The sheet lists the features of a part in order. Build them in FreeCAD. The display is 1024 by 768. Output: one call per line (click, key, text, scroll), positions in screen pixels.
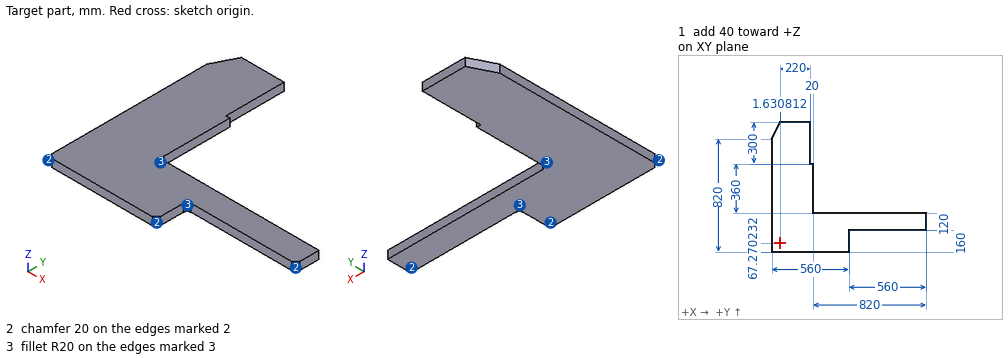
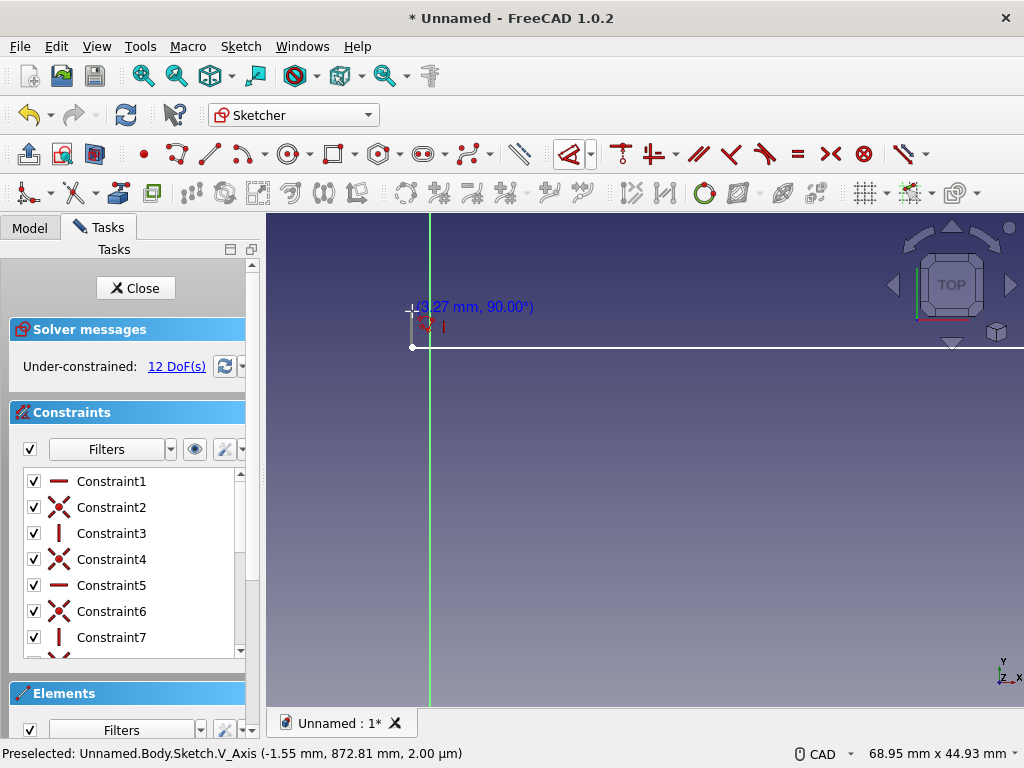
scroll(392, 287, down, 17)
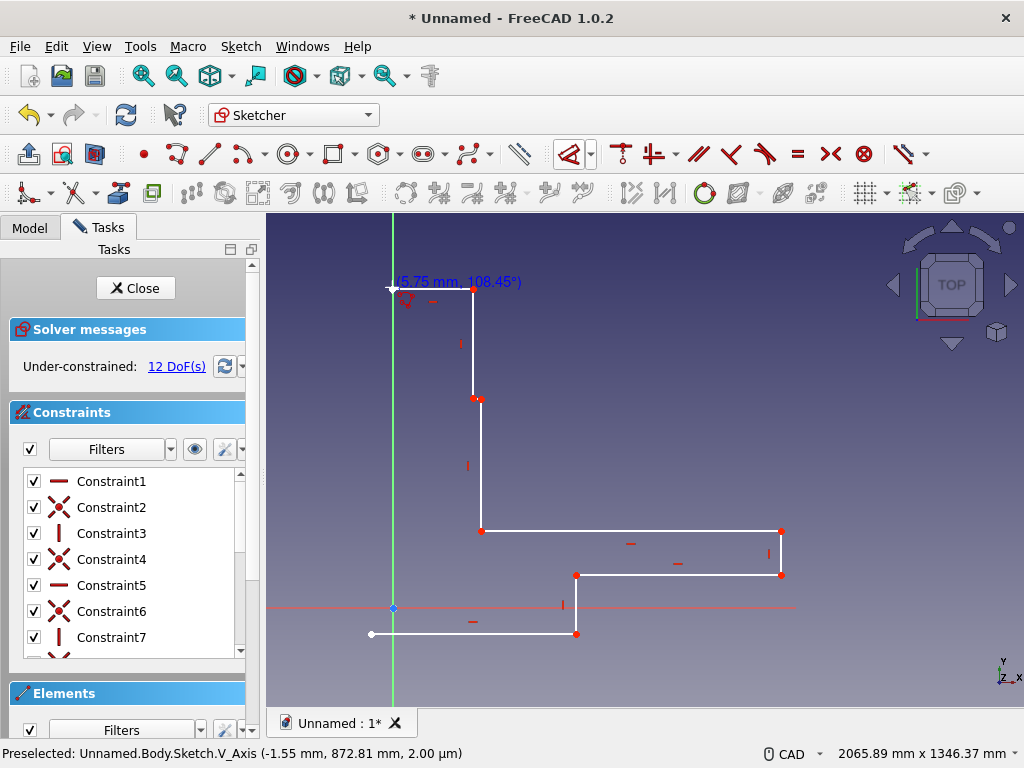
click(371, 332)
click(371, 634)
key(Escape)
key(Escape)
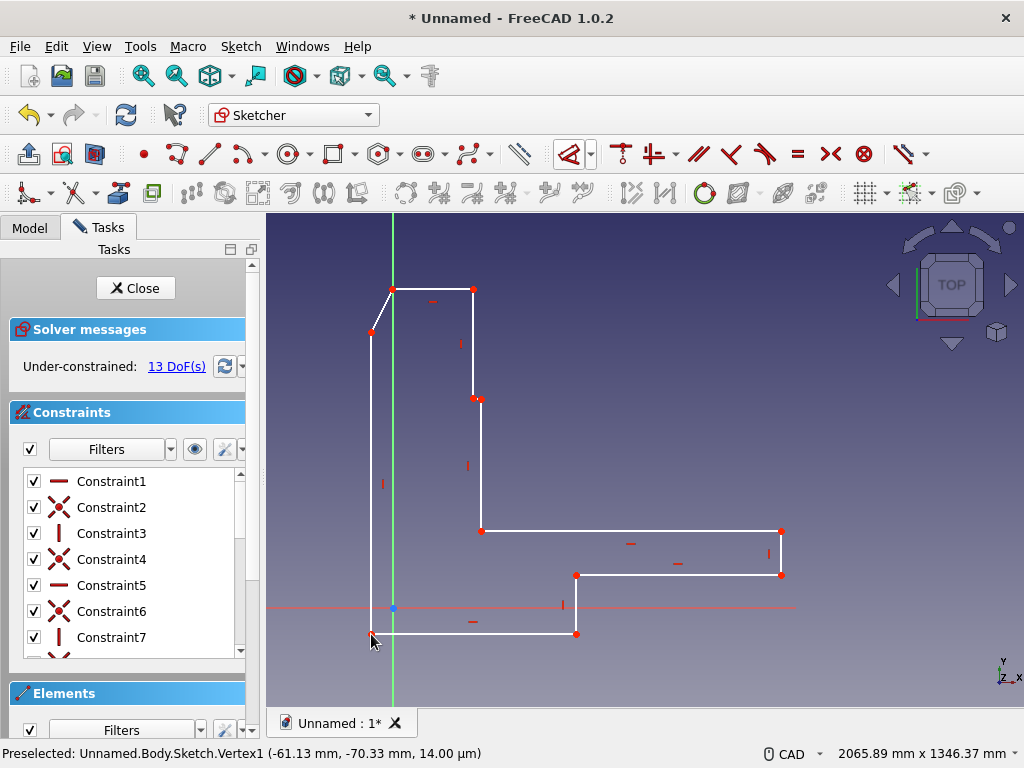
scroll(477, 399, up, 7)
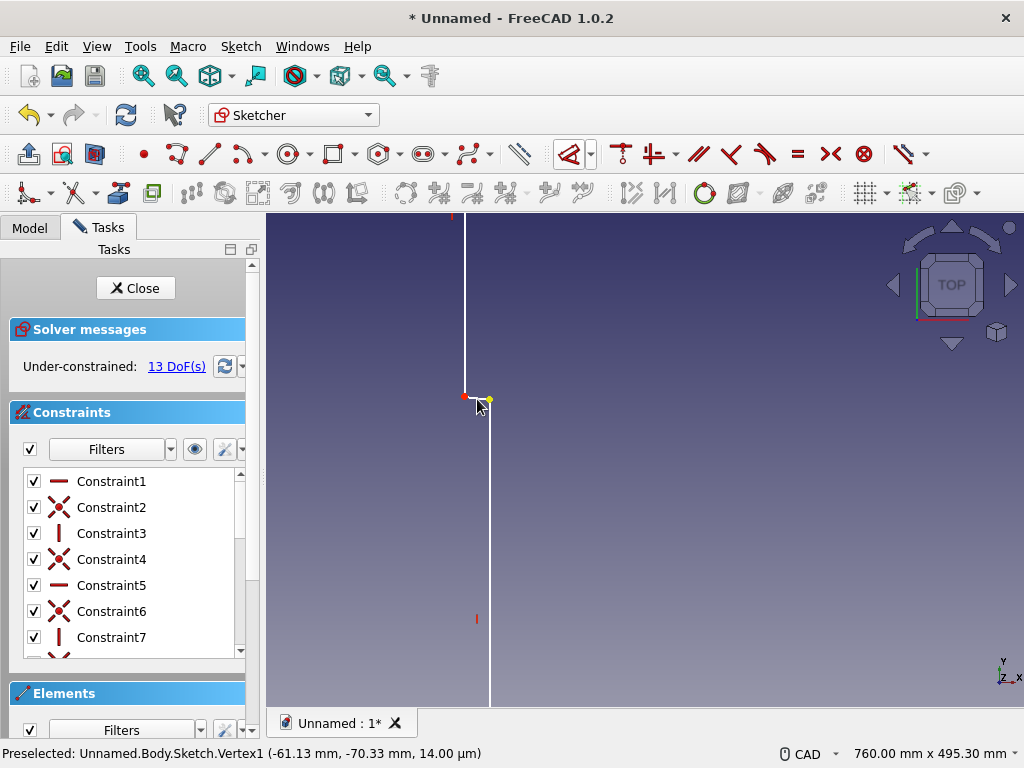
click(477, 398)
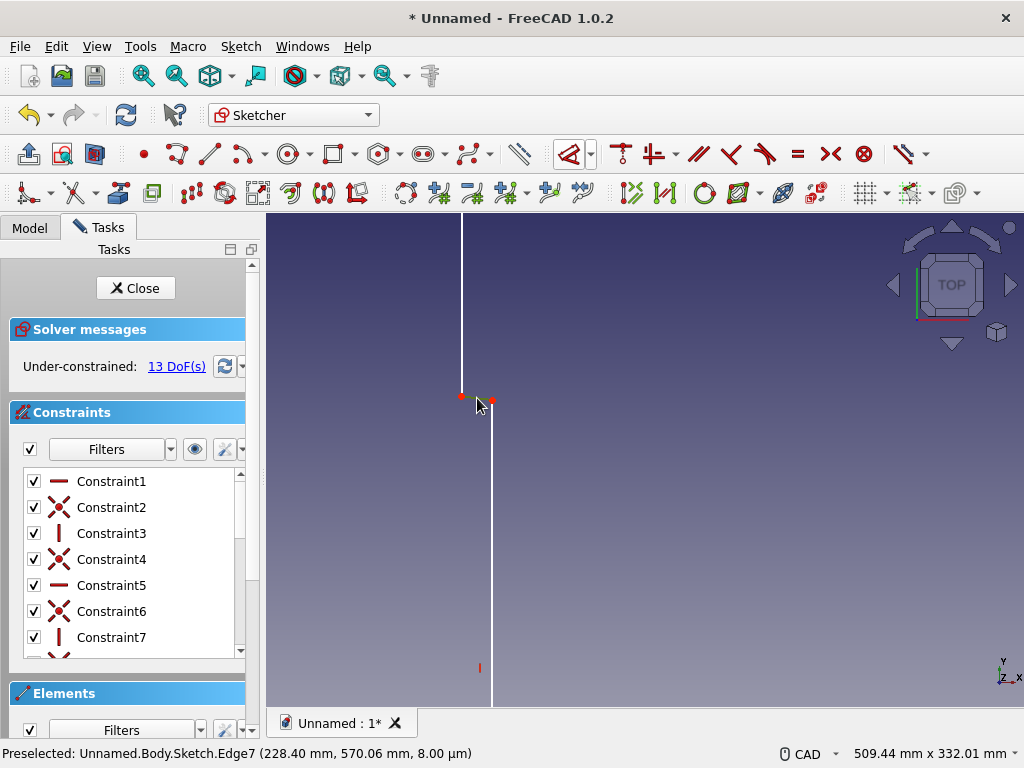
key(h)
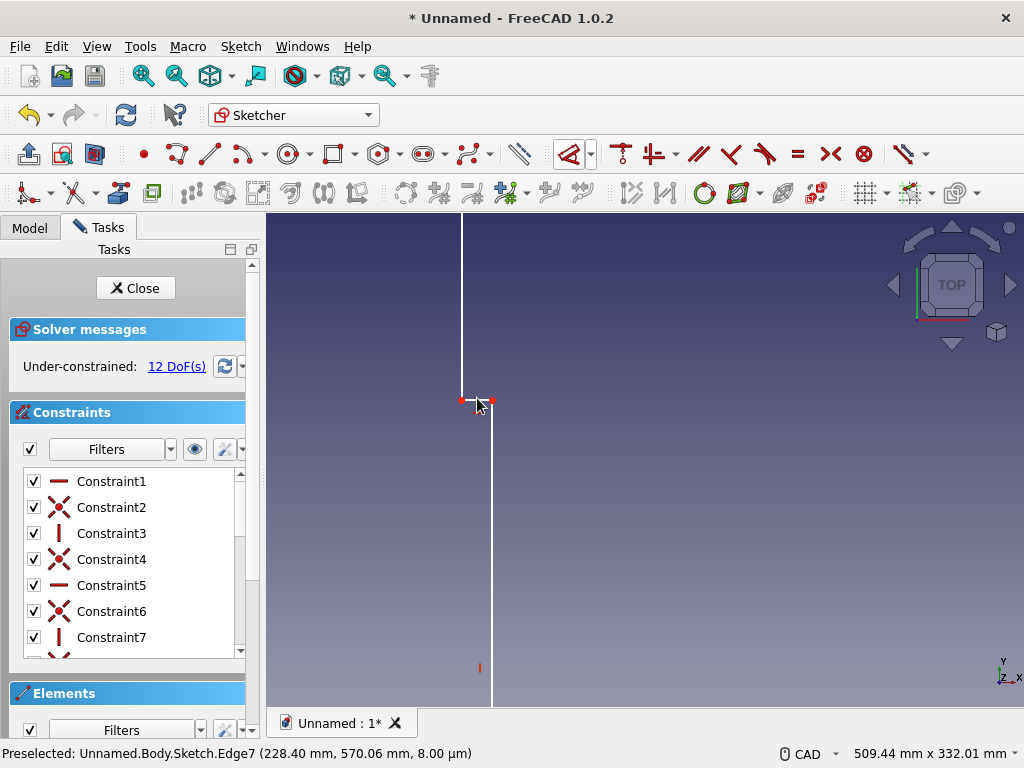
key(d)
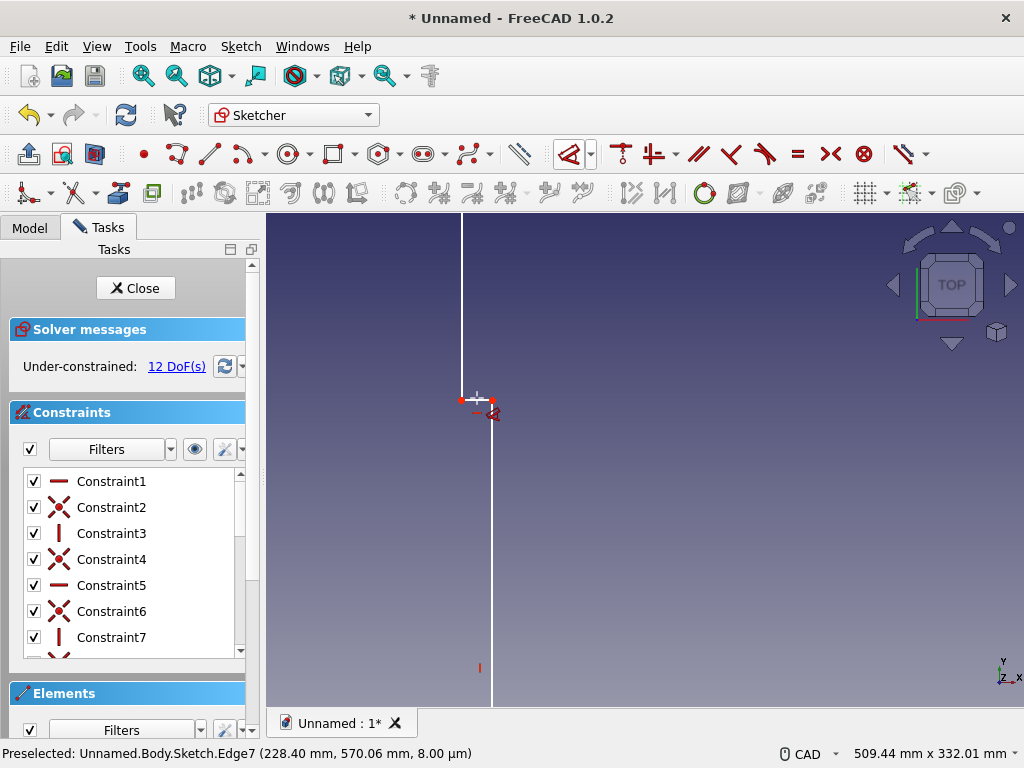
scroll(483, 400, up, 3)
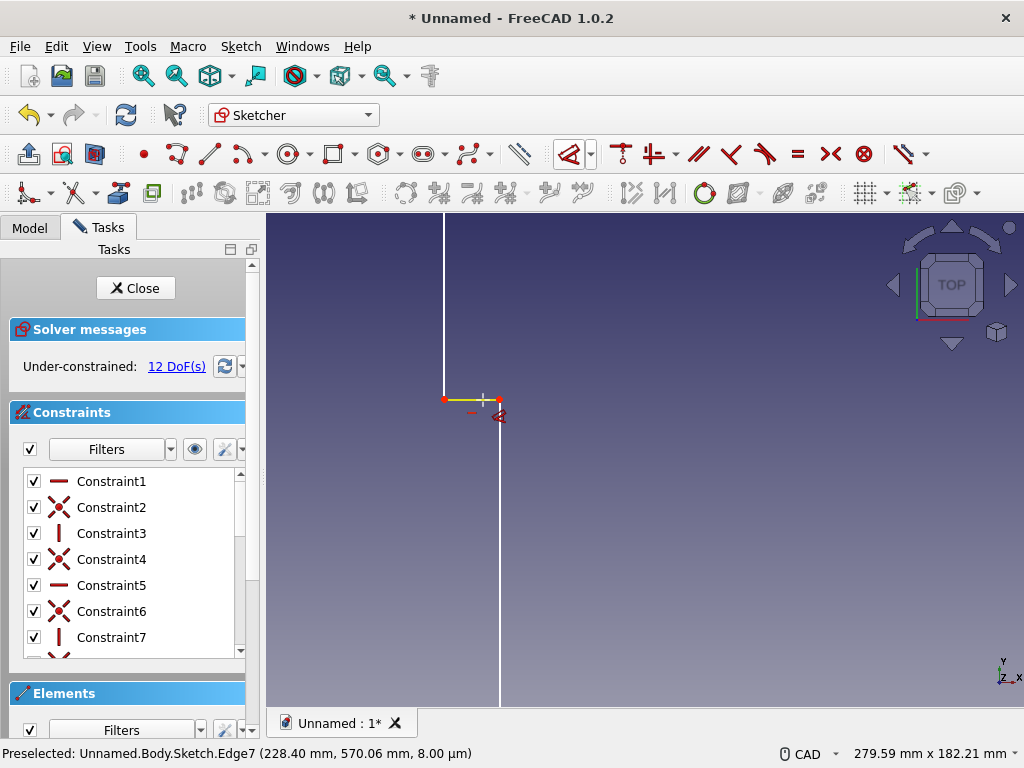
click(483, 400)
click(472, 366)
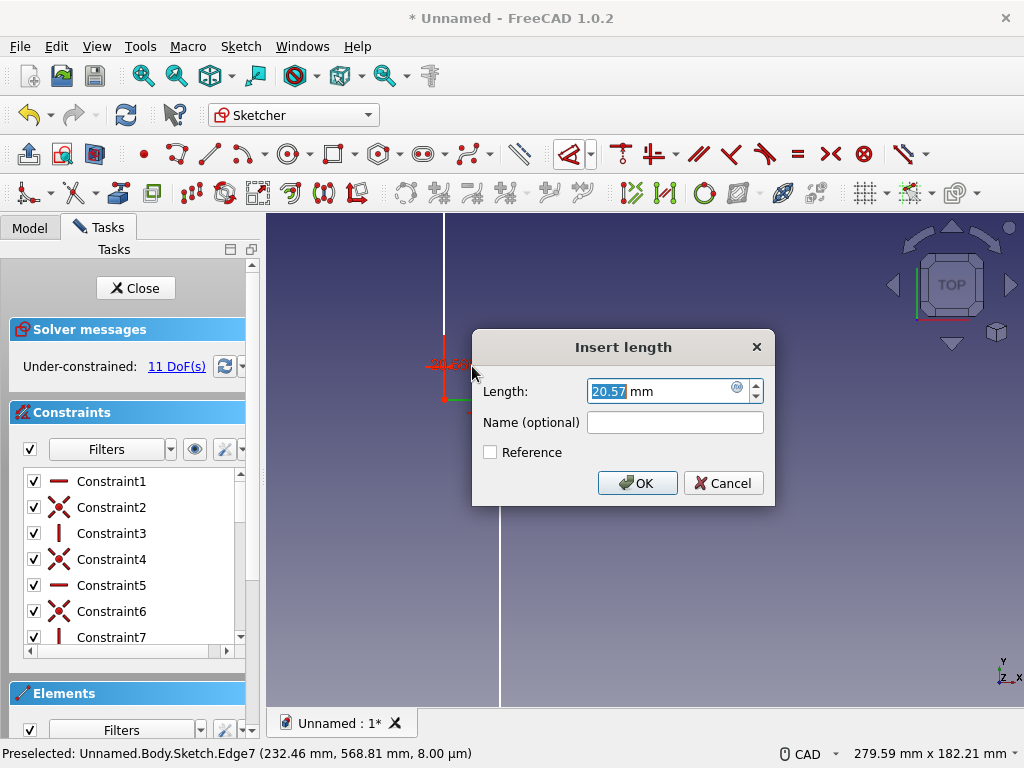
text(20)
key(Return)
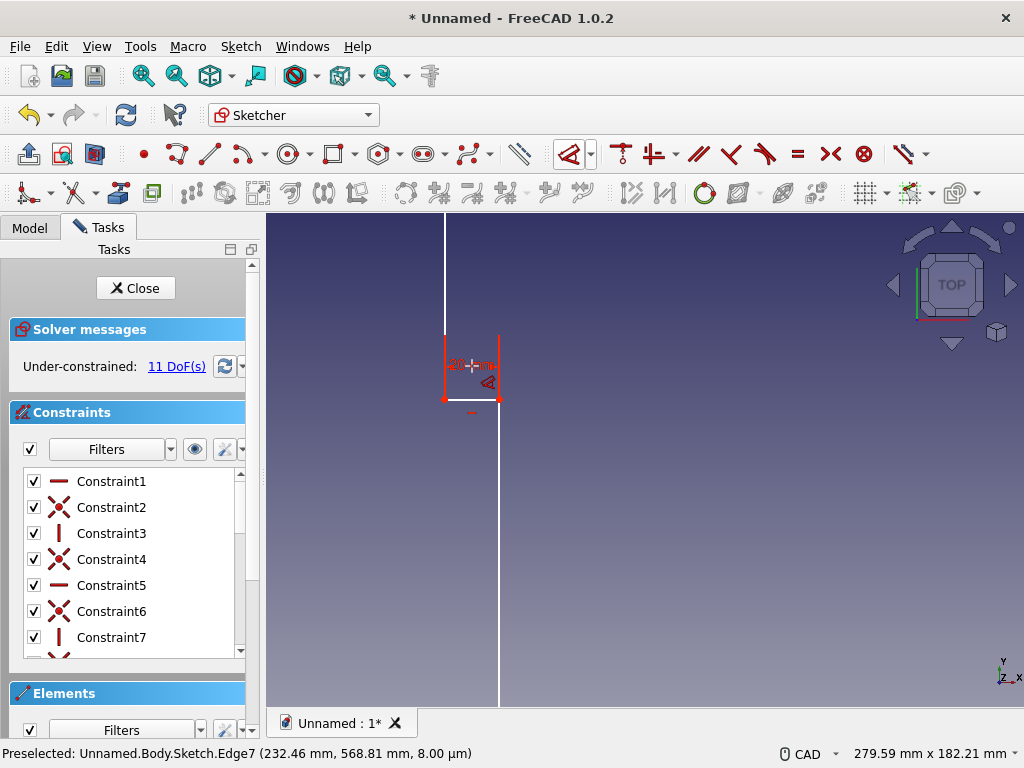
scroll(498, 411, down, 11)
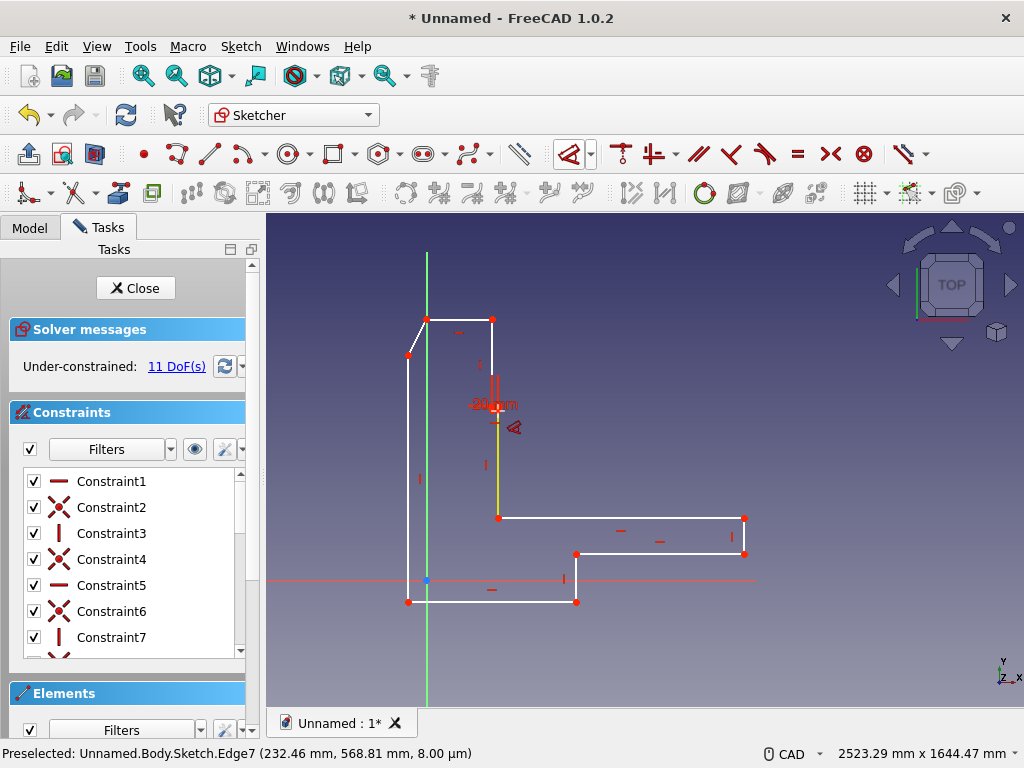
click(459, 602)
click(492, 636)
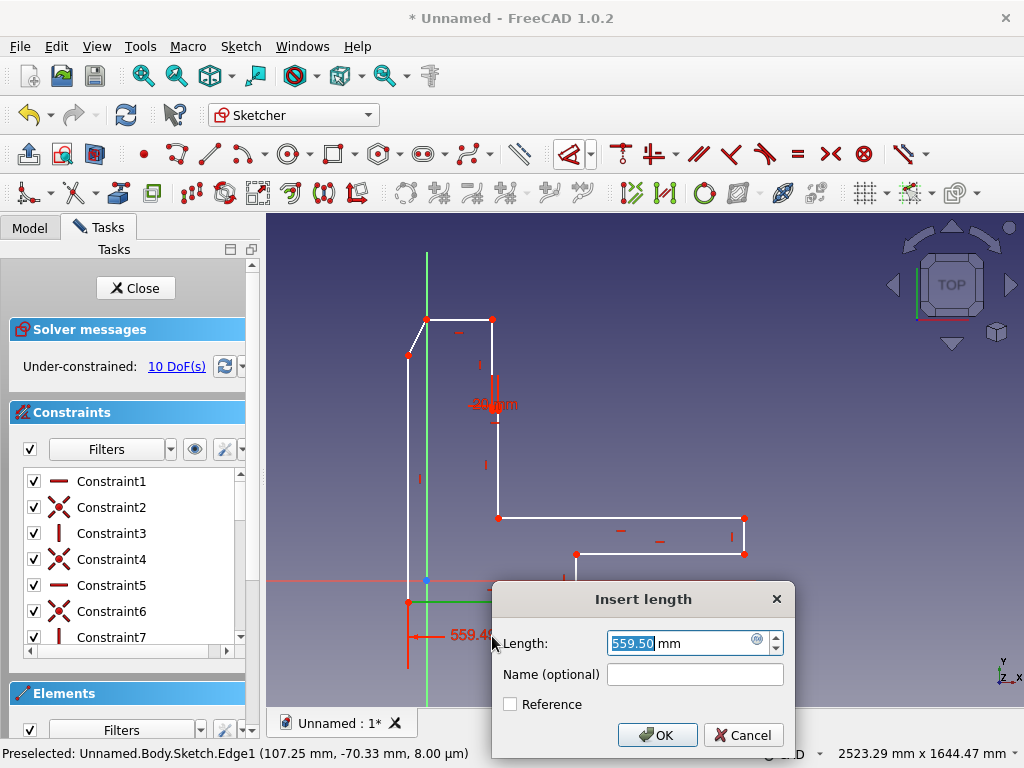
text(560)
key(Return)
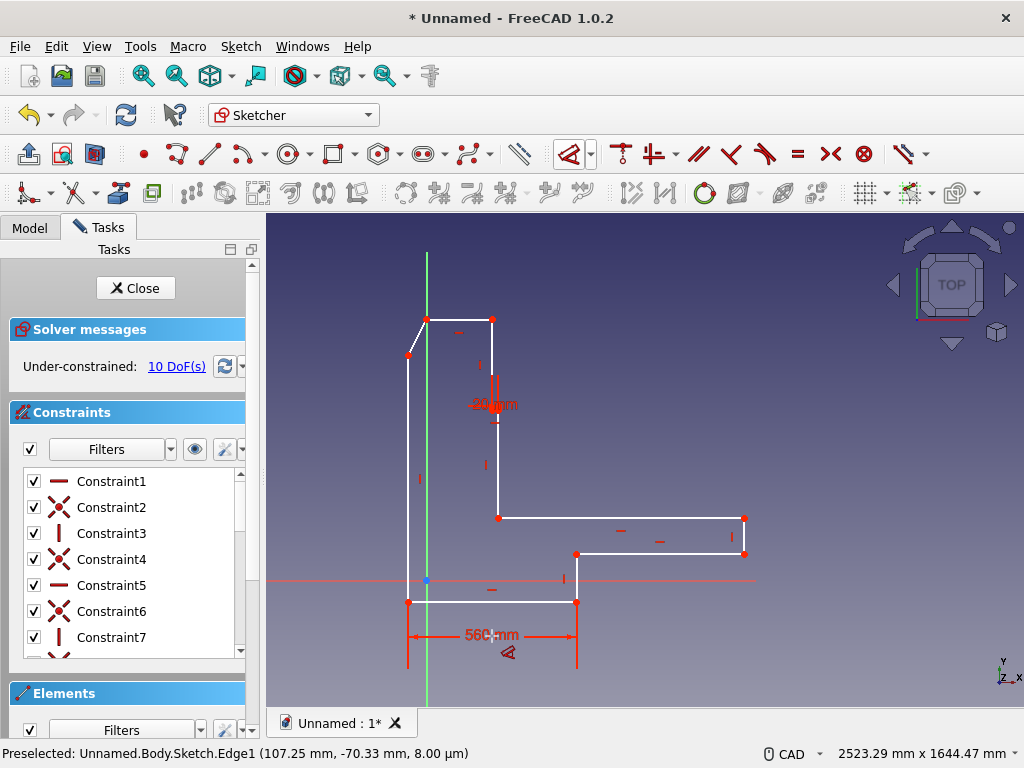
click(577, 569)
click(611, 595)